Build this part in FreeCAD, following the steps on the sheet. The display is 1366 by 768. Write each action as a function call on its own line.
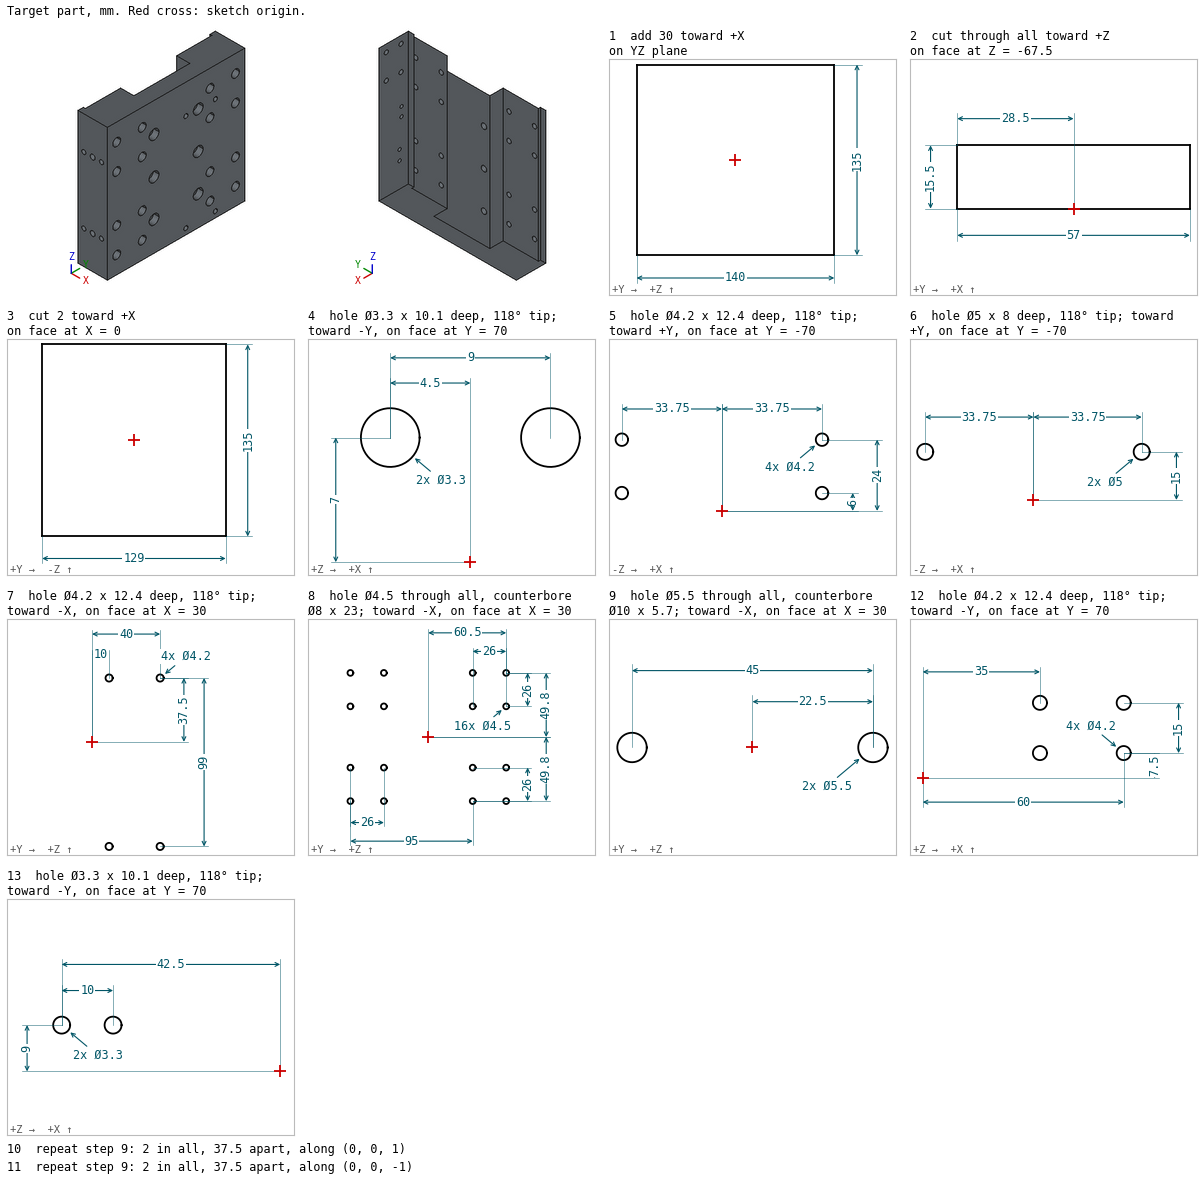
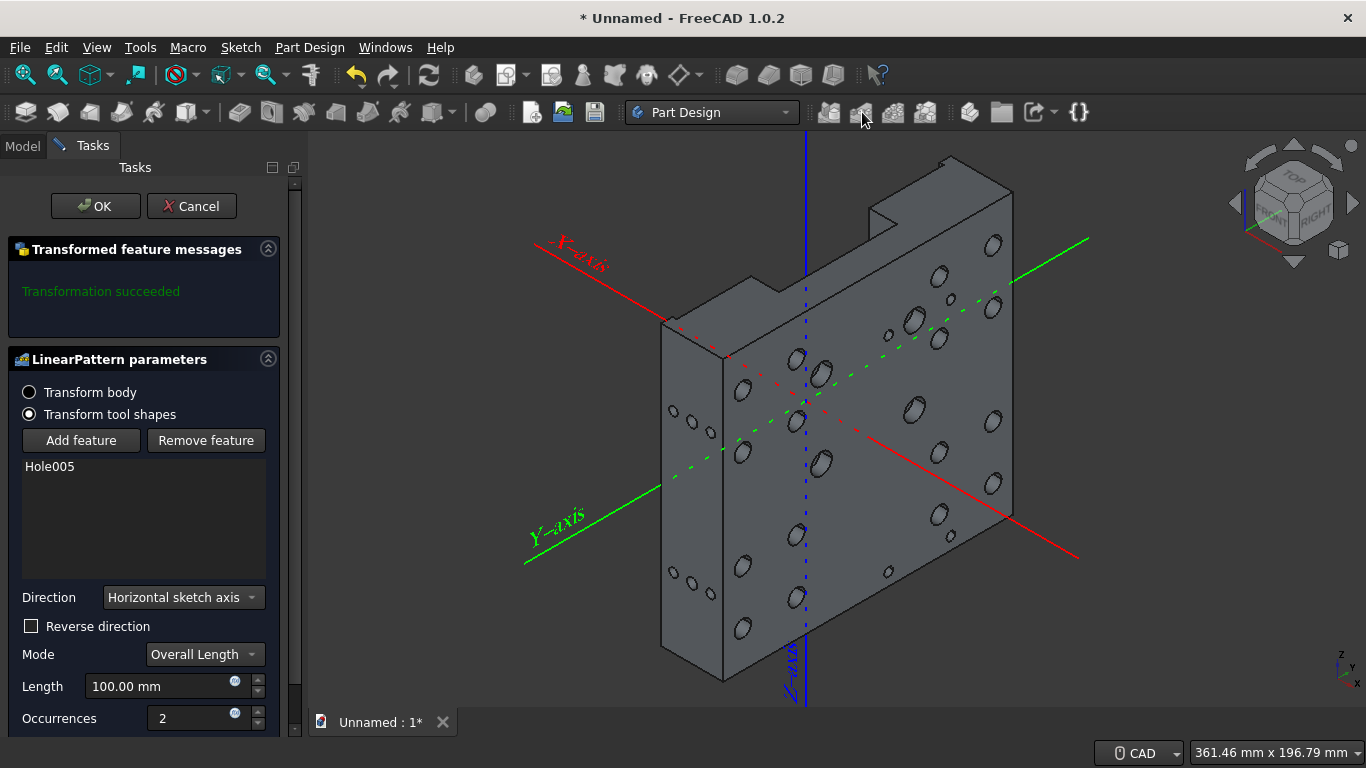
click(184, 598)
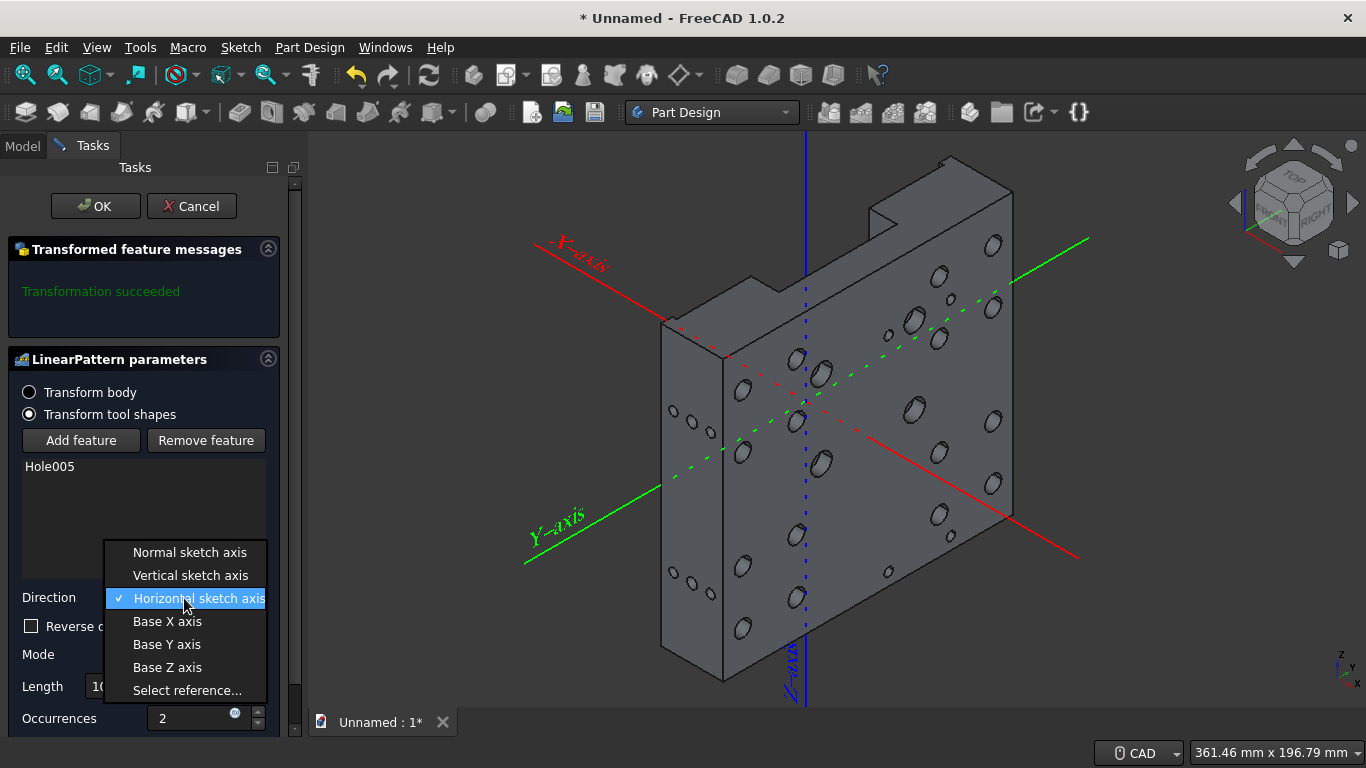
click(184, 668)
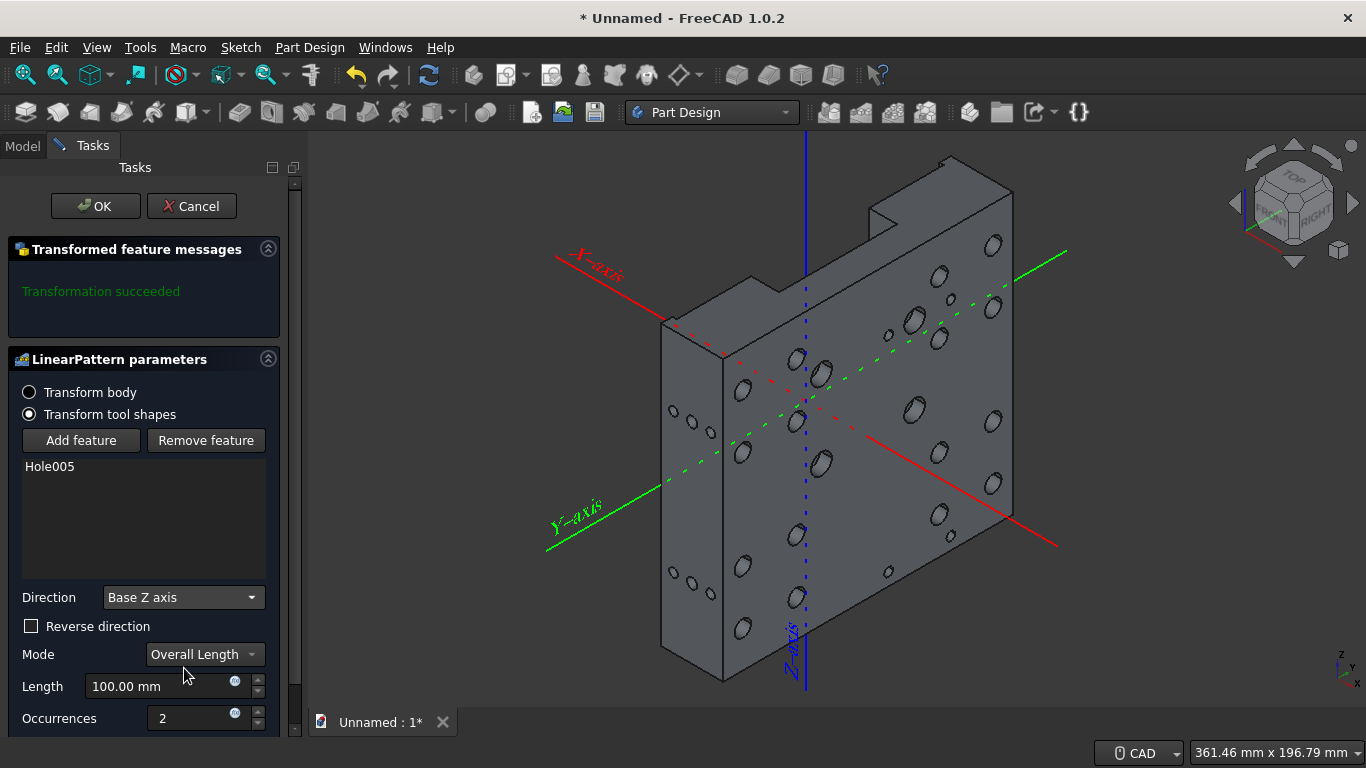
click(206, 654)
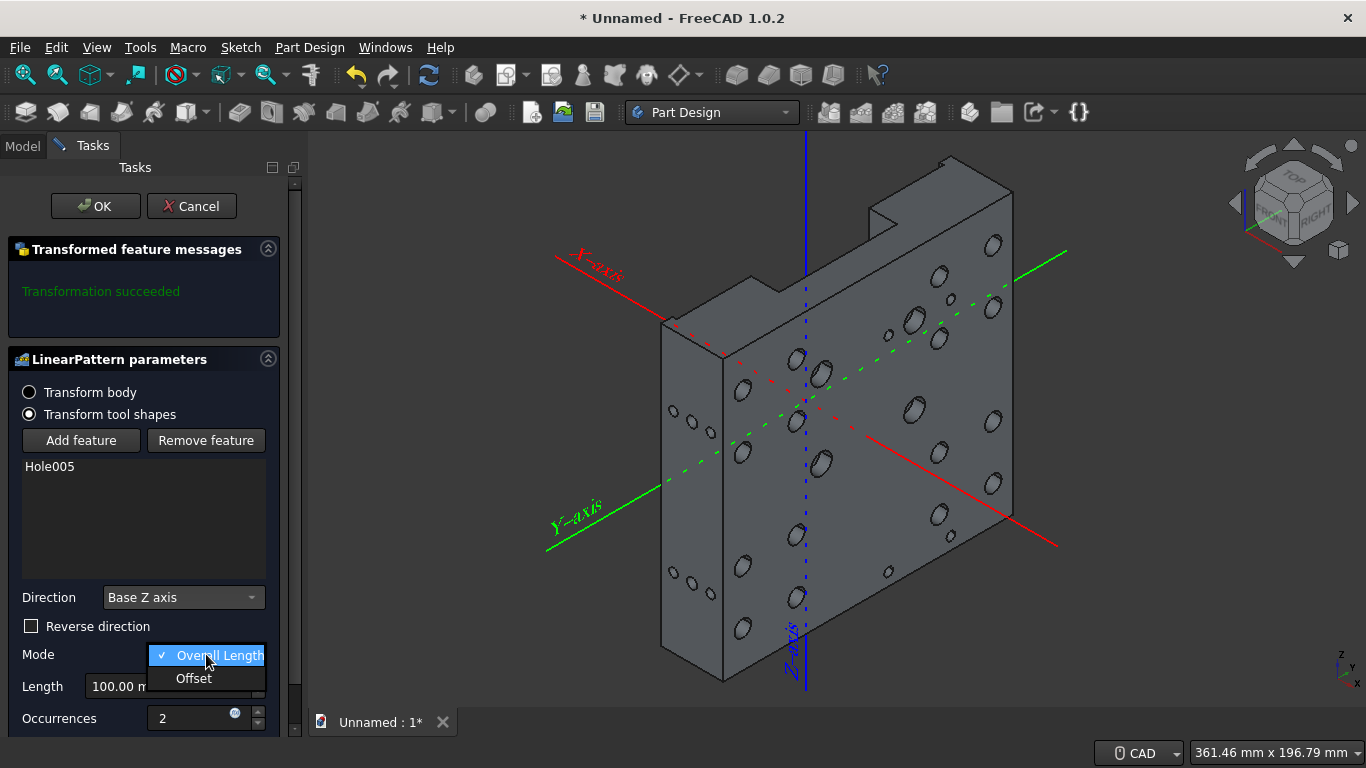
click(206, 678)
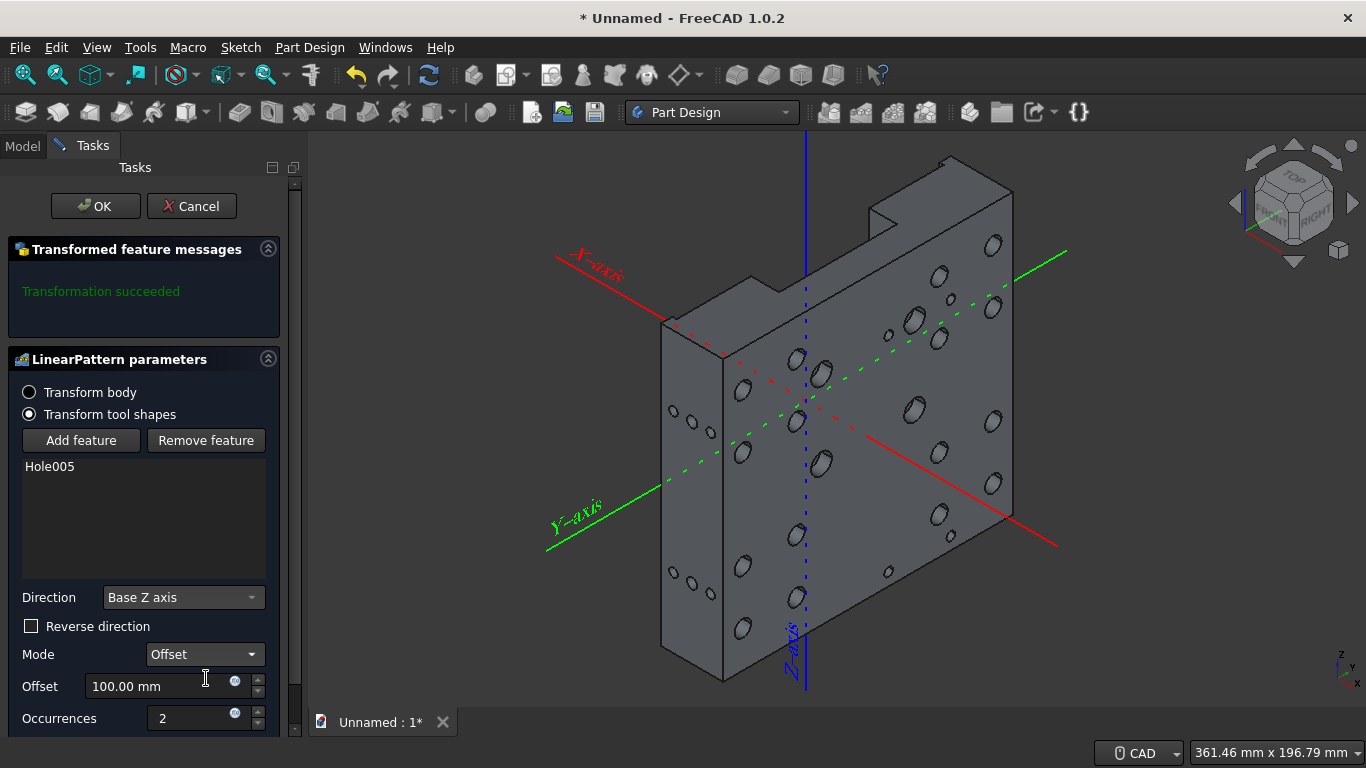
triple_click(168, 686)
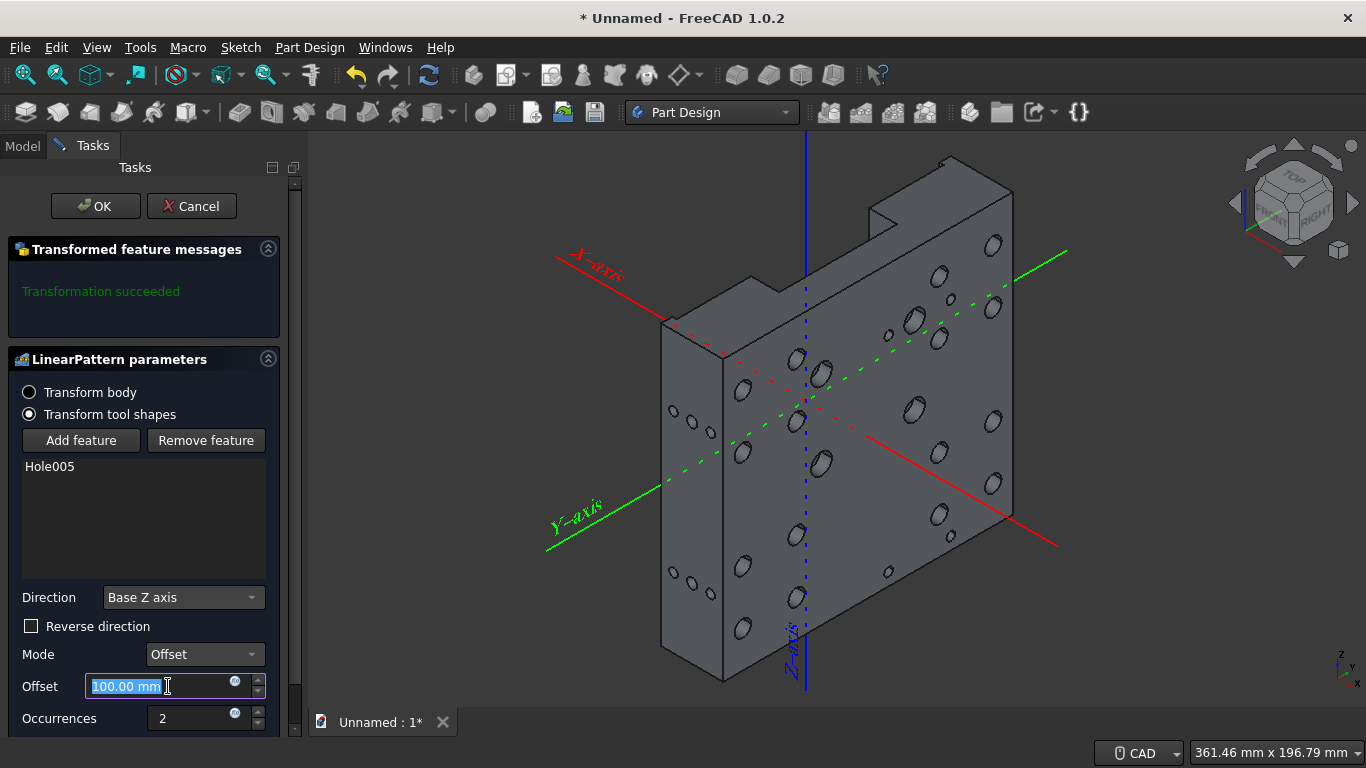
text(37.5)
key(Tab)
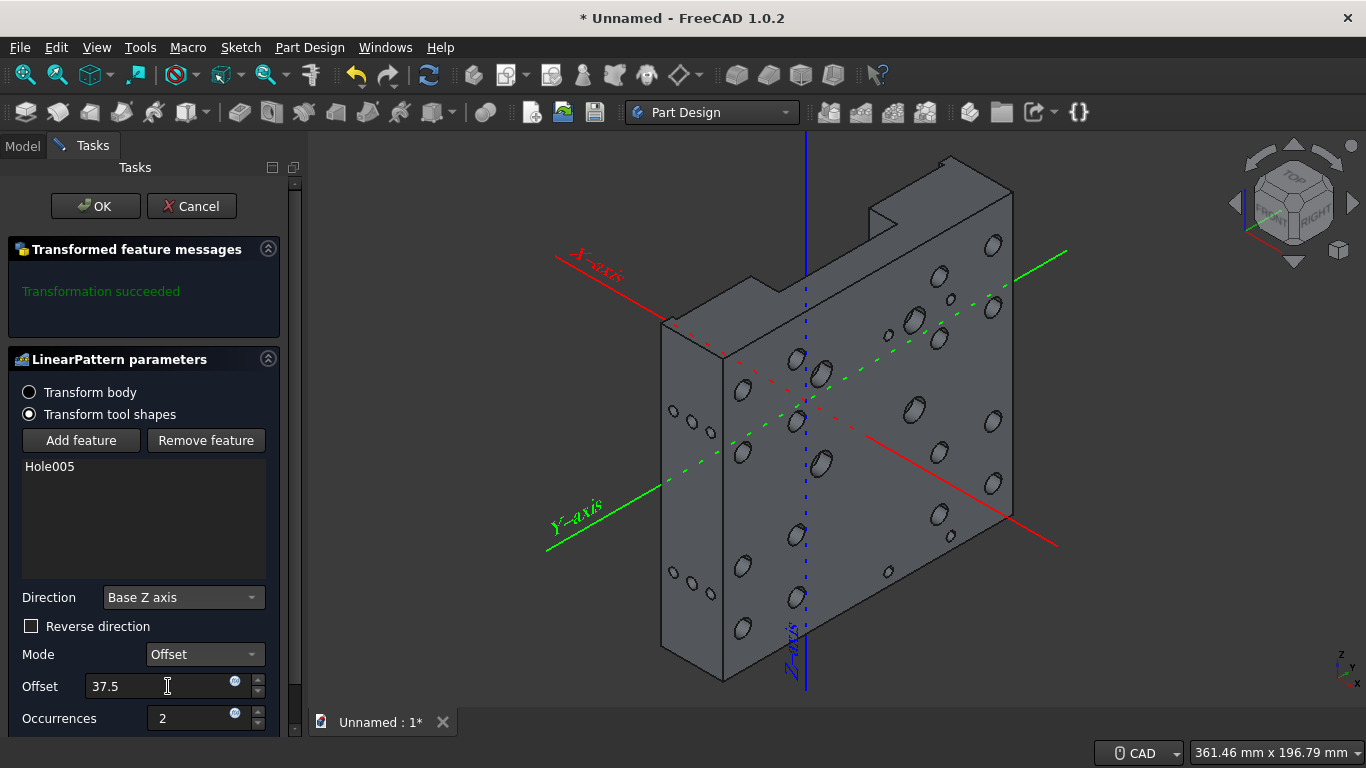
triple_click(198, 718)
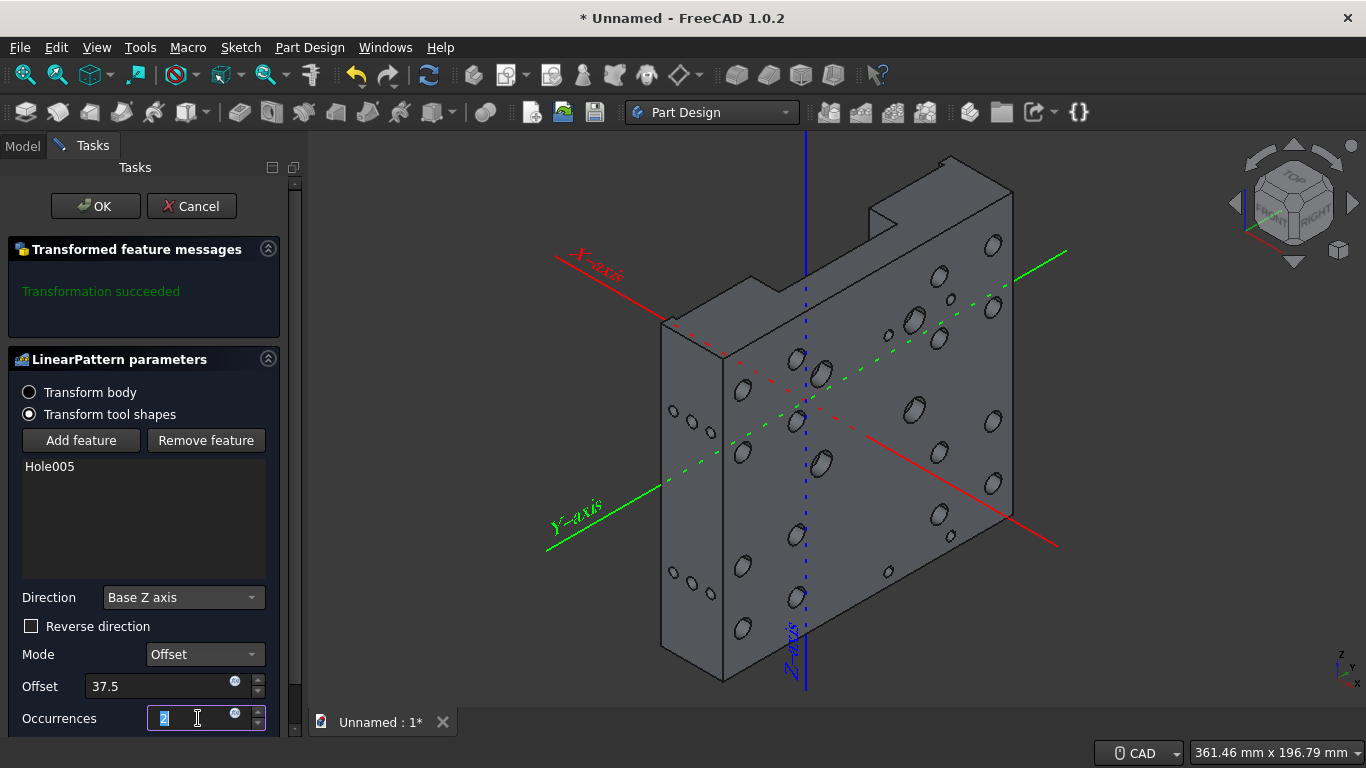
text(2)
key(Tab)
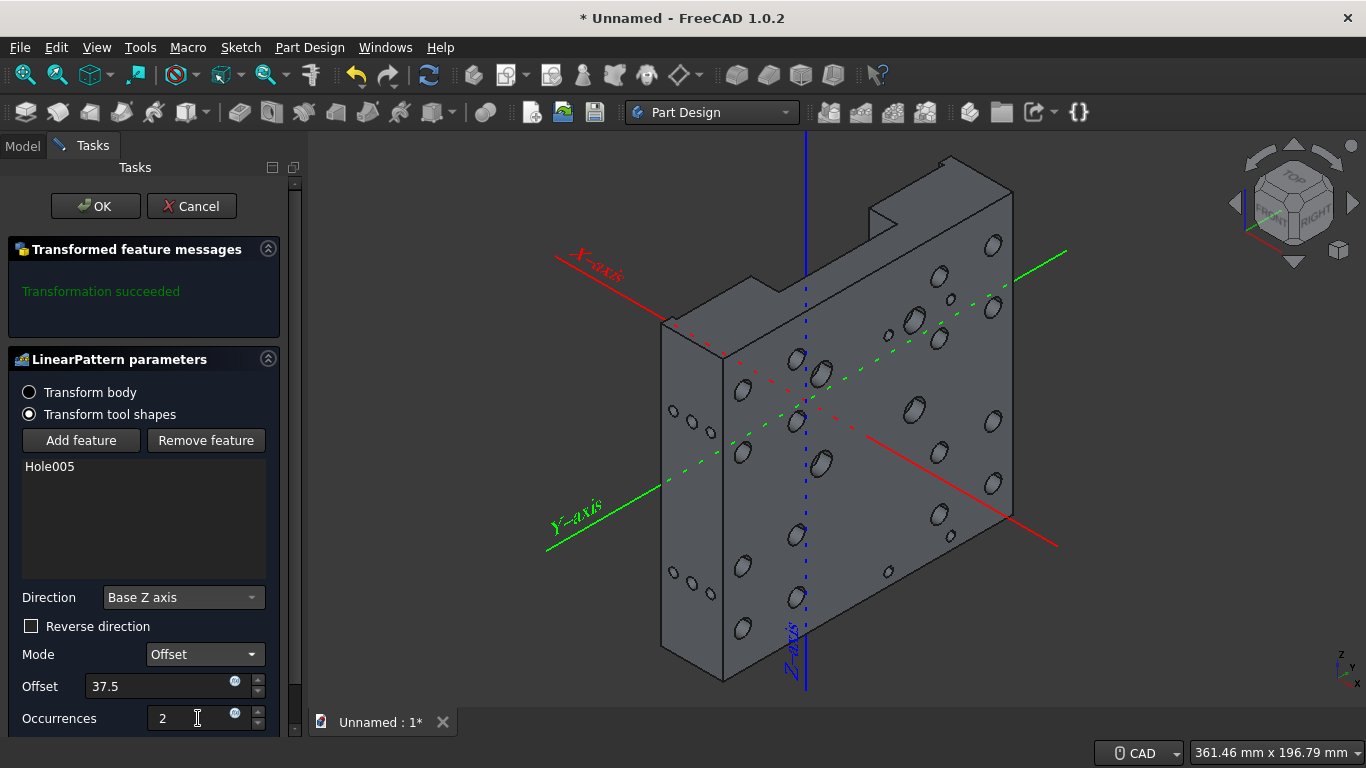
click(30, 626)